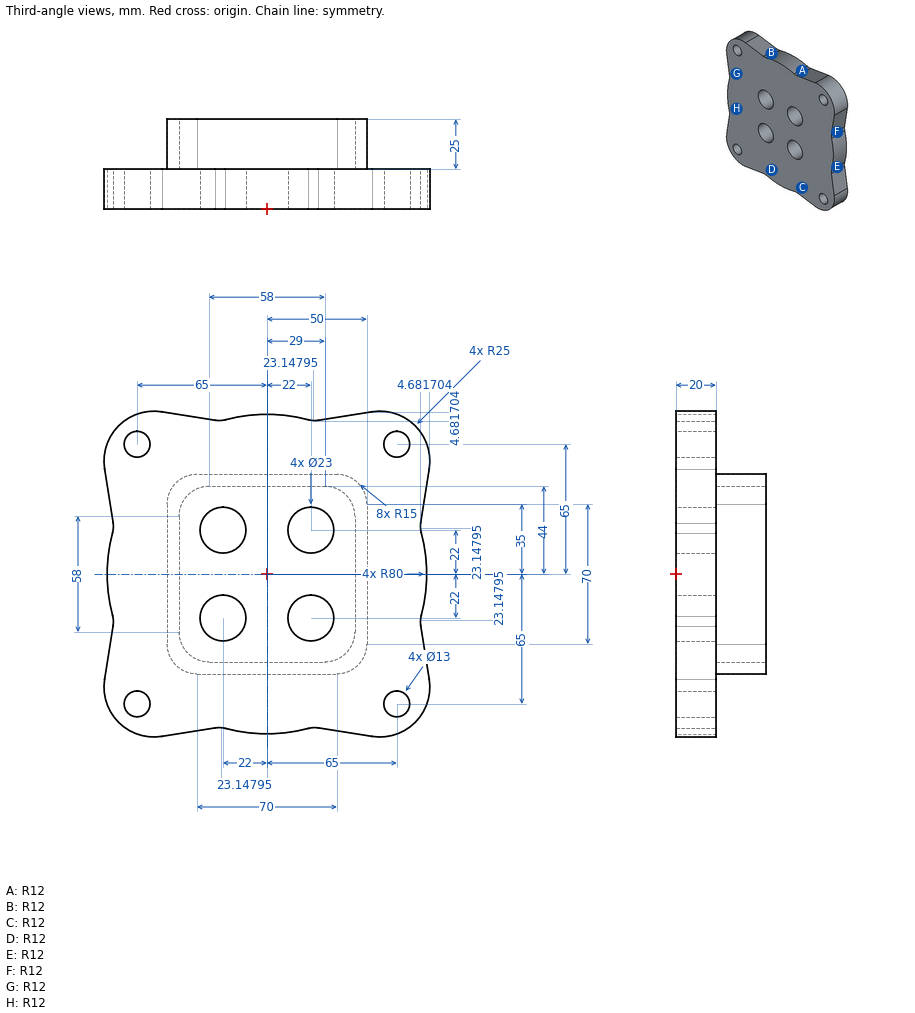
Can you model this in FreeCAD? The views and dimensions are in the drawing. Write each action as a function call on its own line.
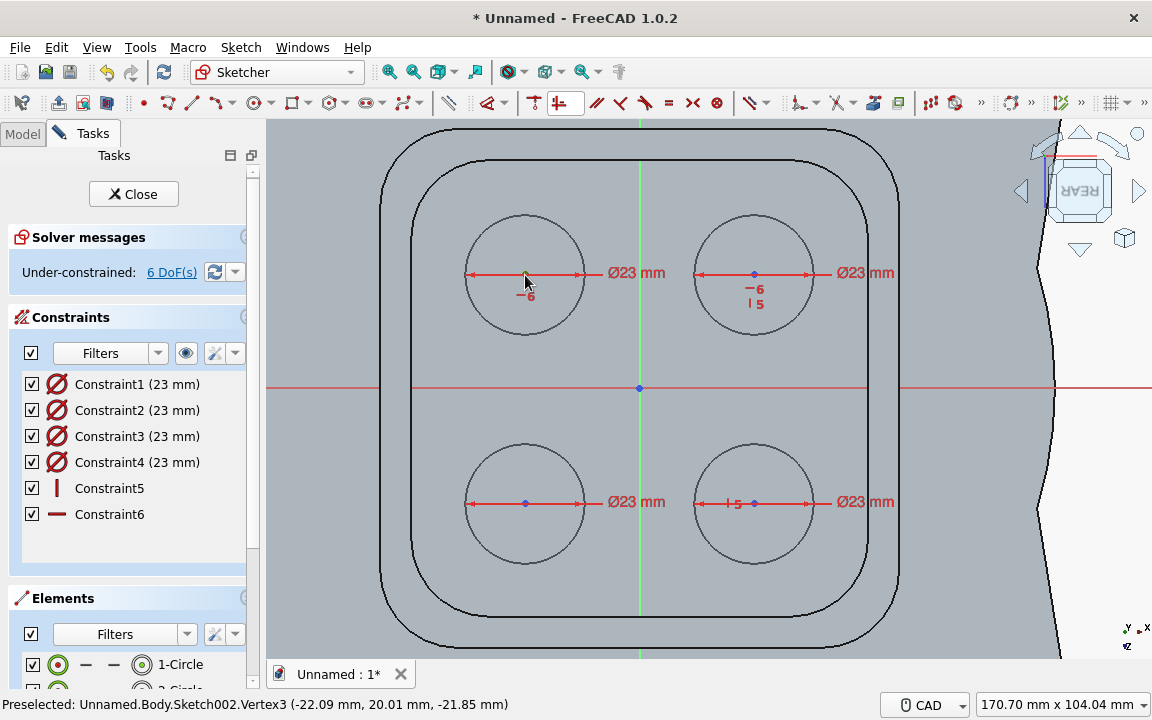
click(525, 504)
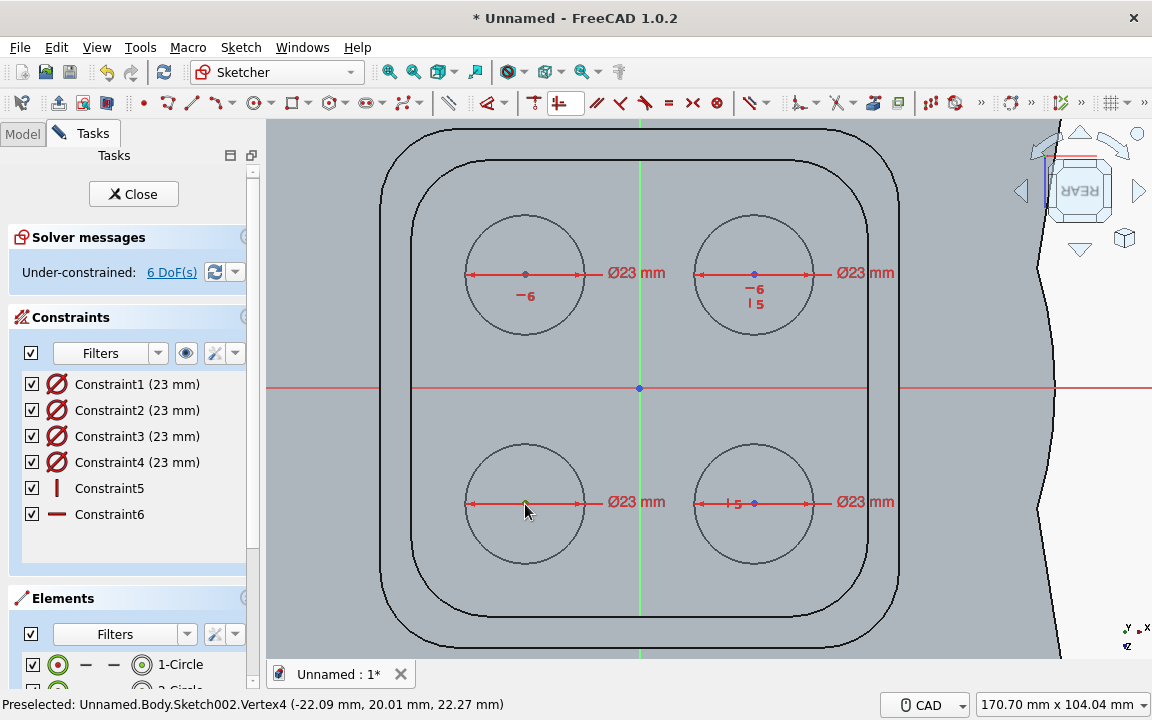
click(578, 104)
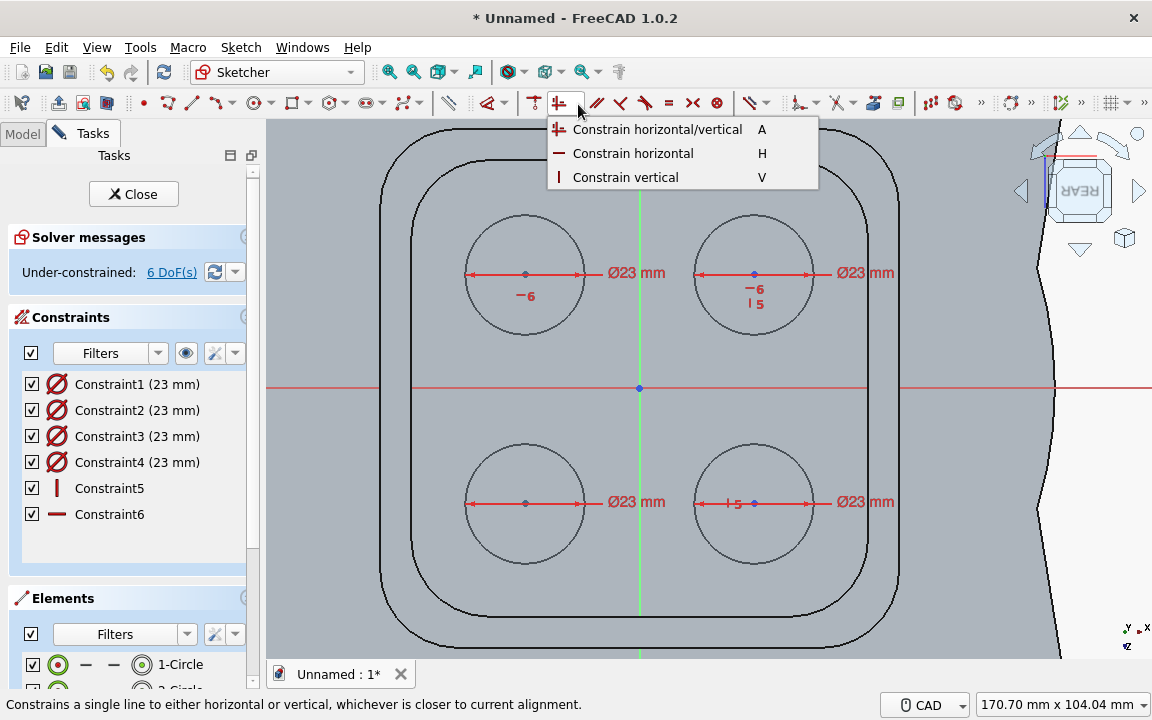
click(683, 177)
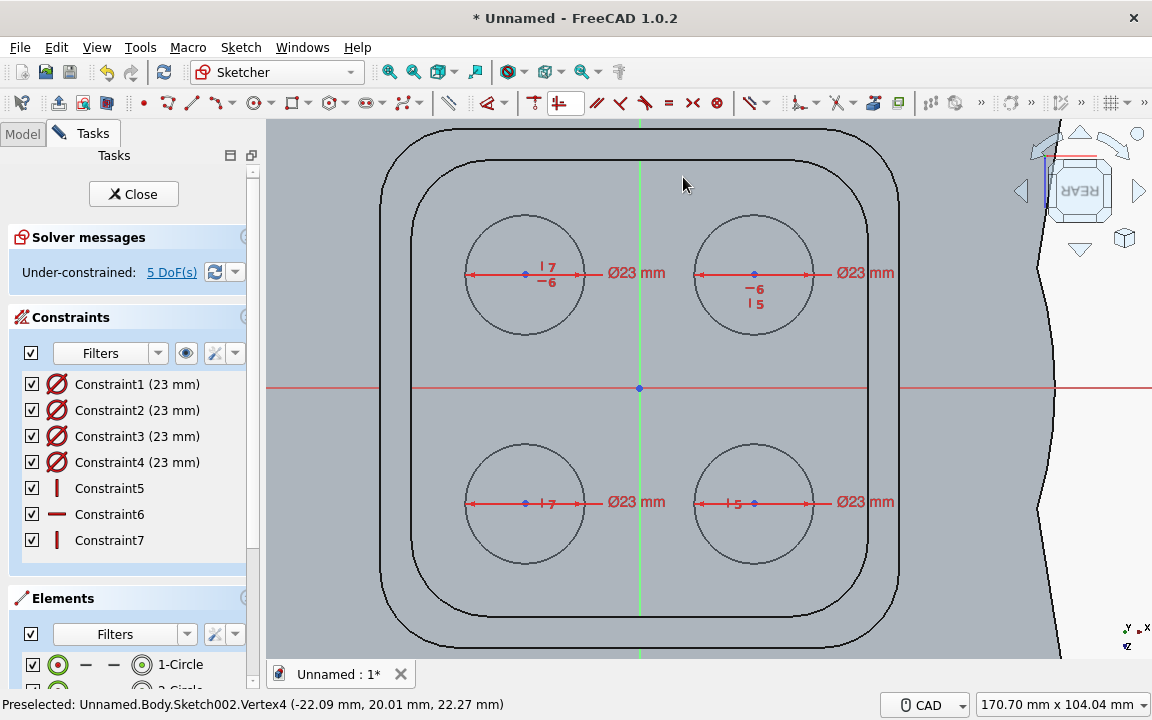
click(754, 504)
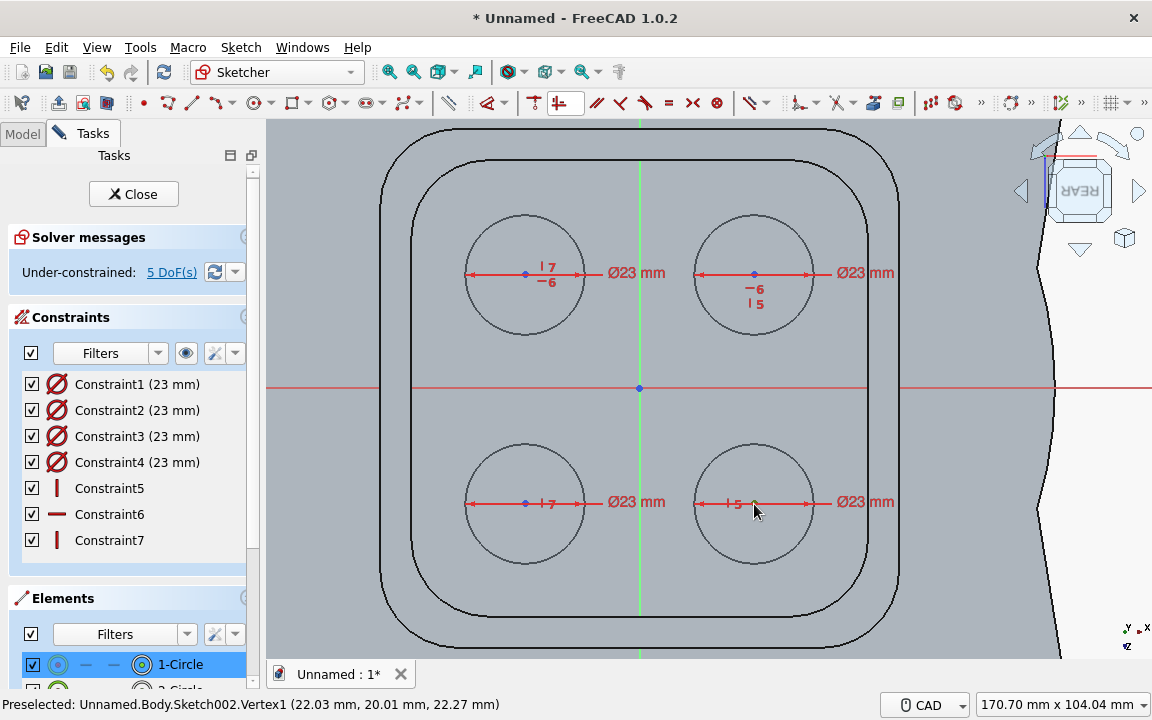
click(525, 504)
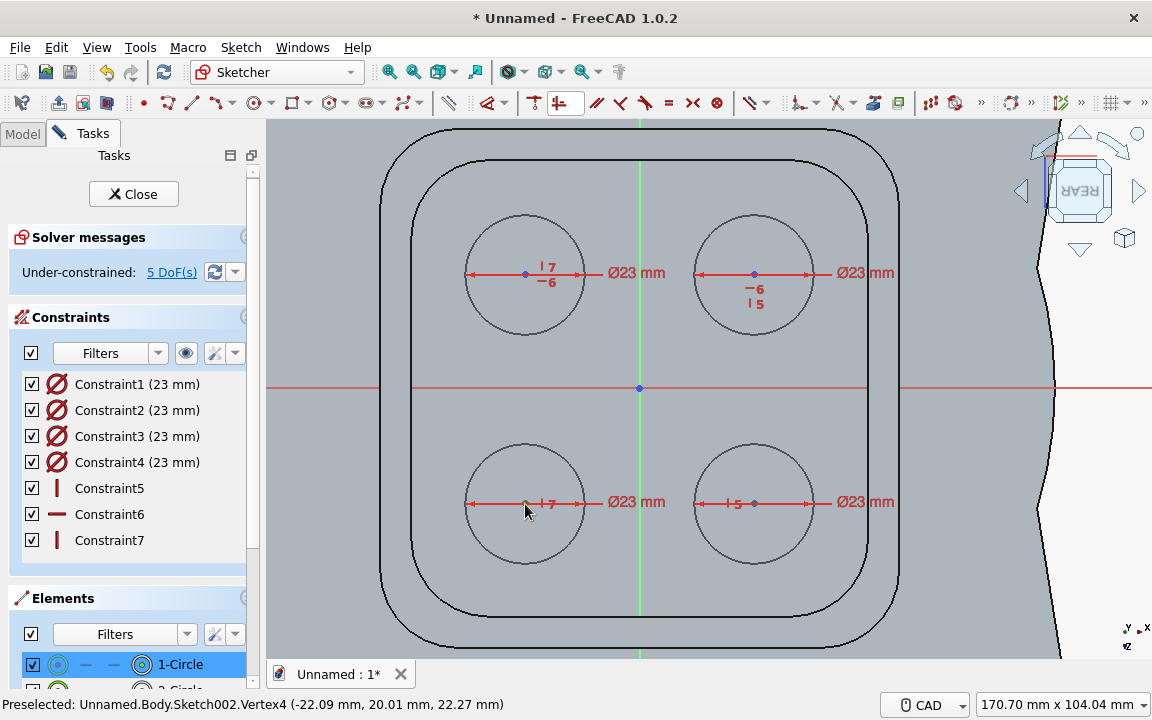
click(578, 104)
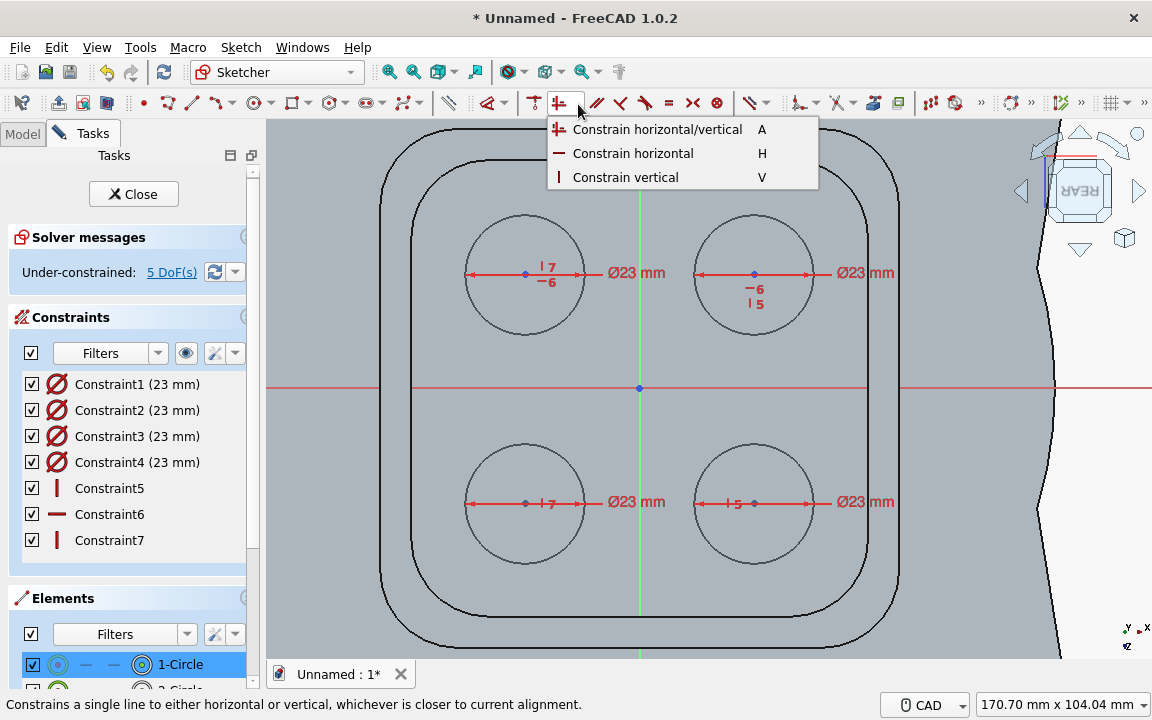
click(683, 153)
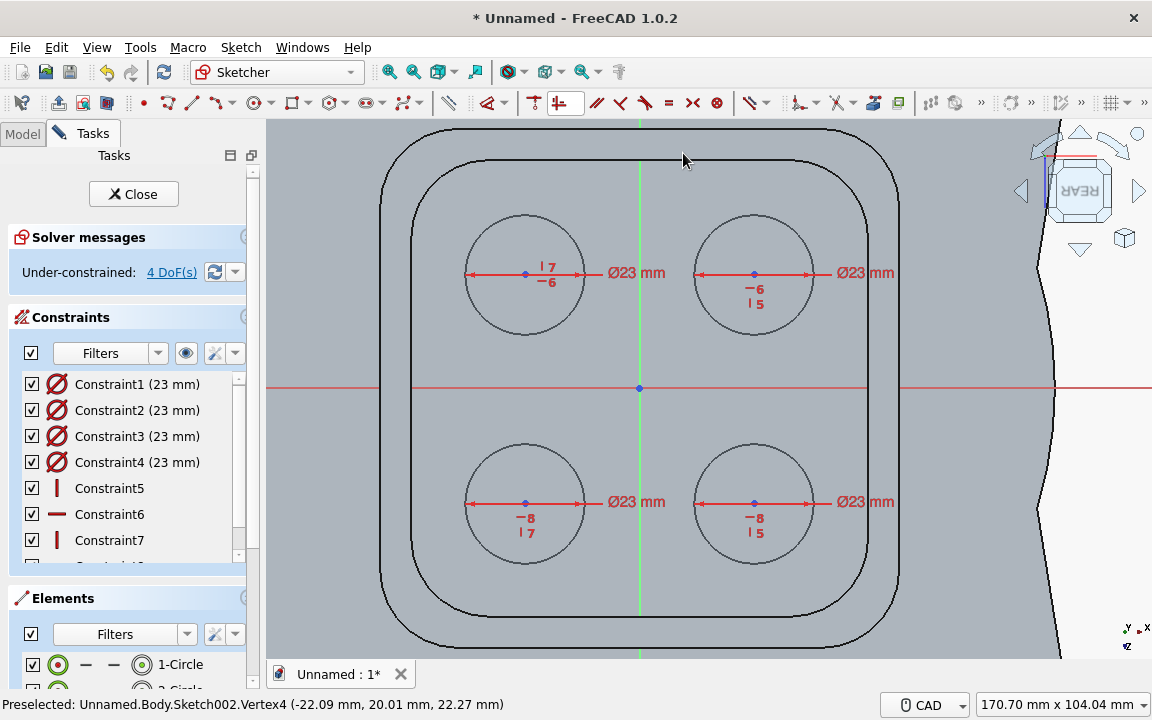
click(488, 104)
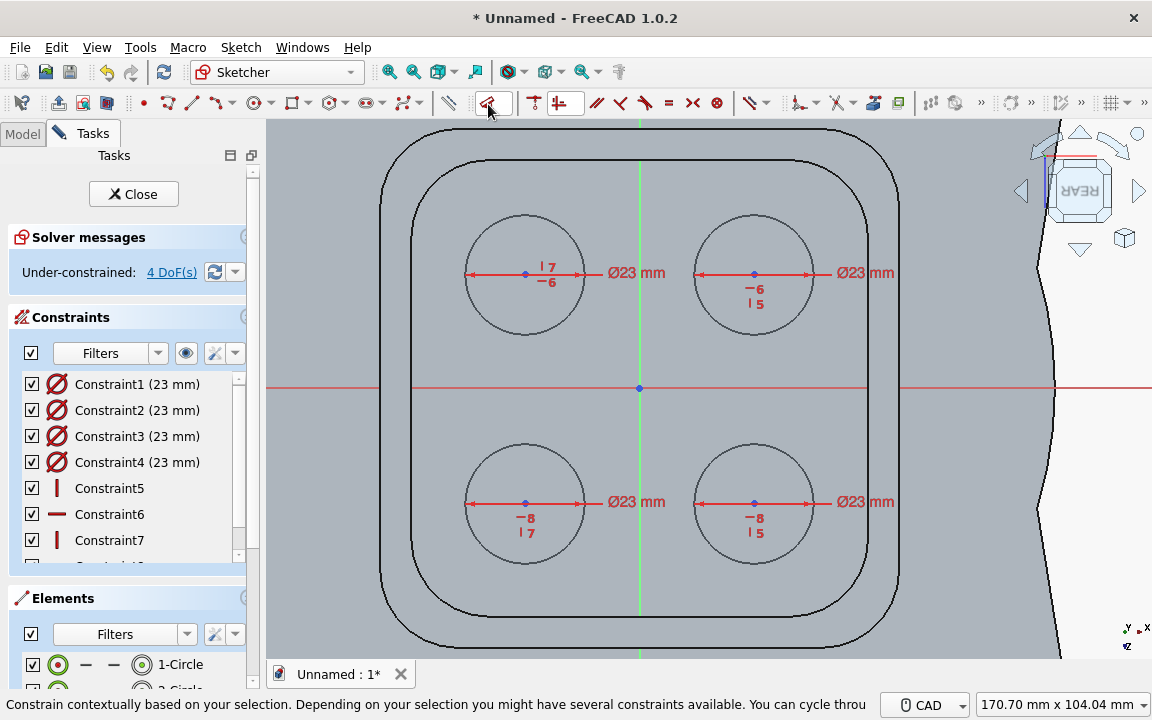
click(754, 504)
click(671, 538)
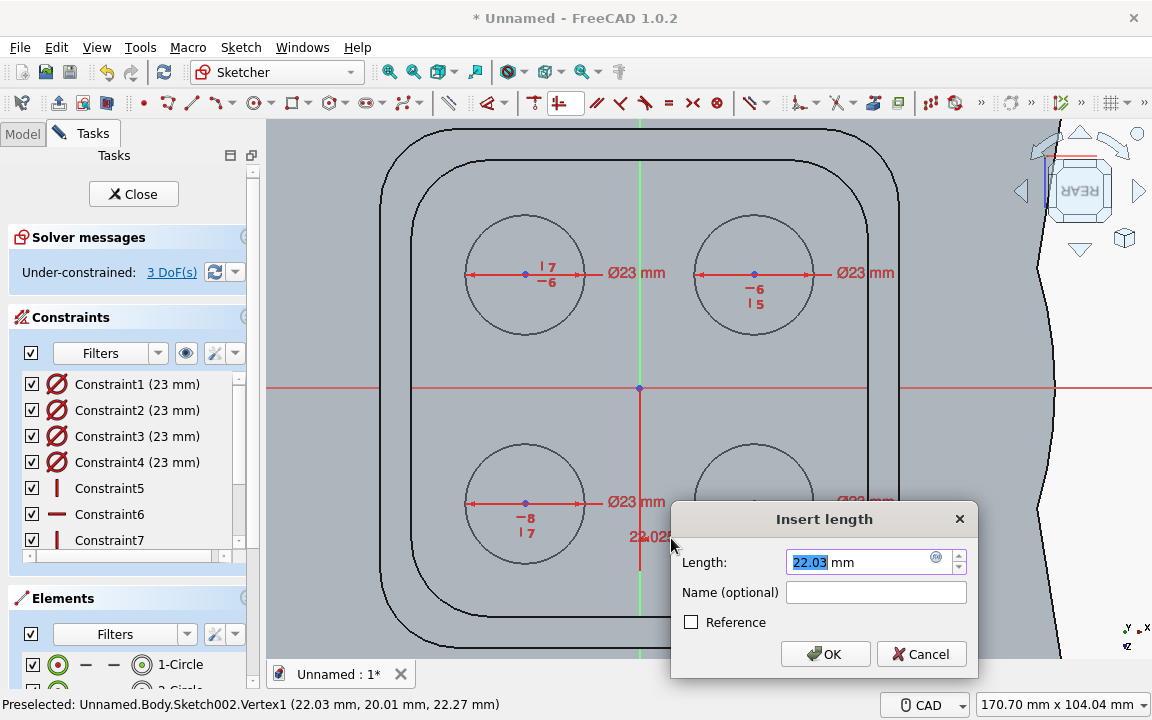
text(22)
key(Return)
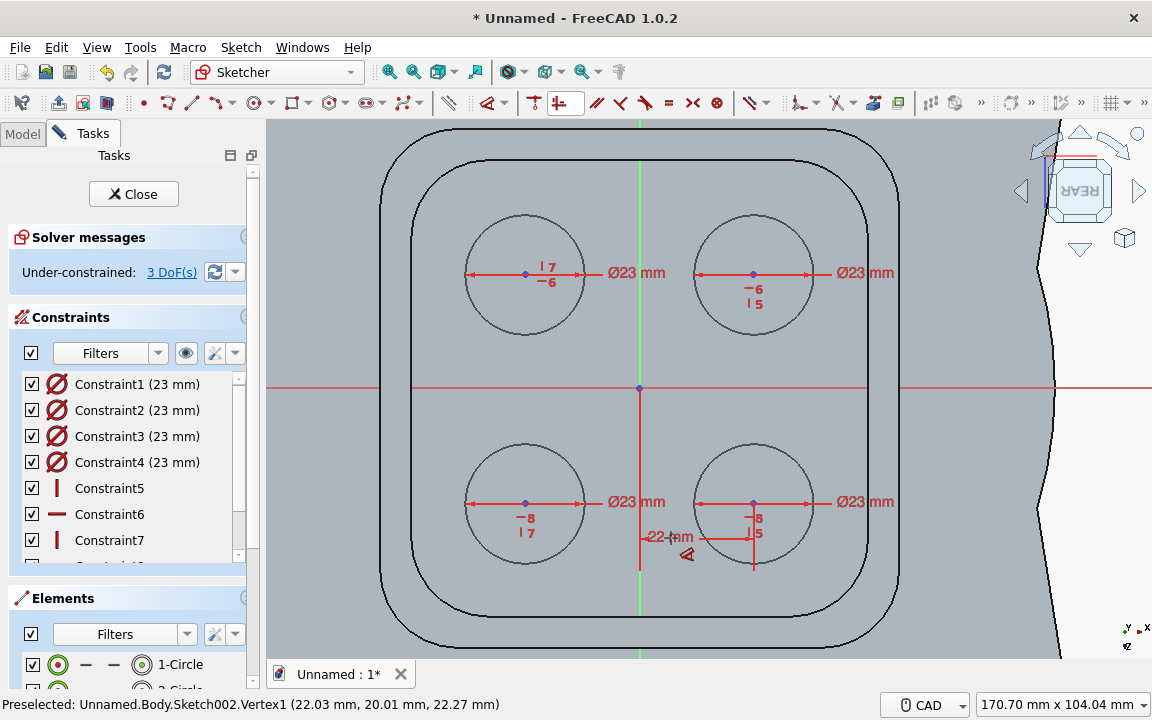
click(754, 504)
click(788, 420)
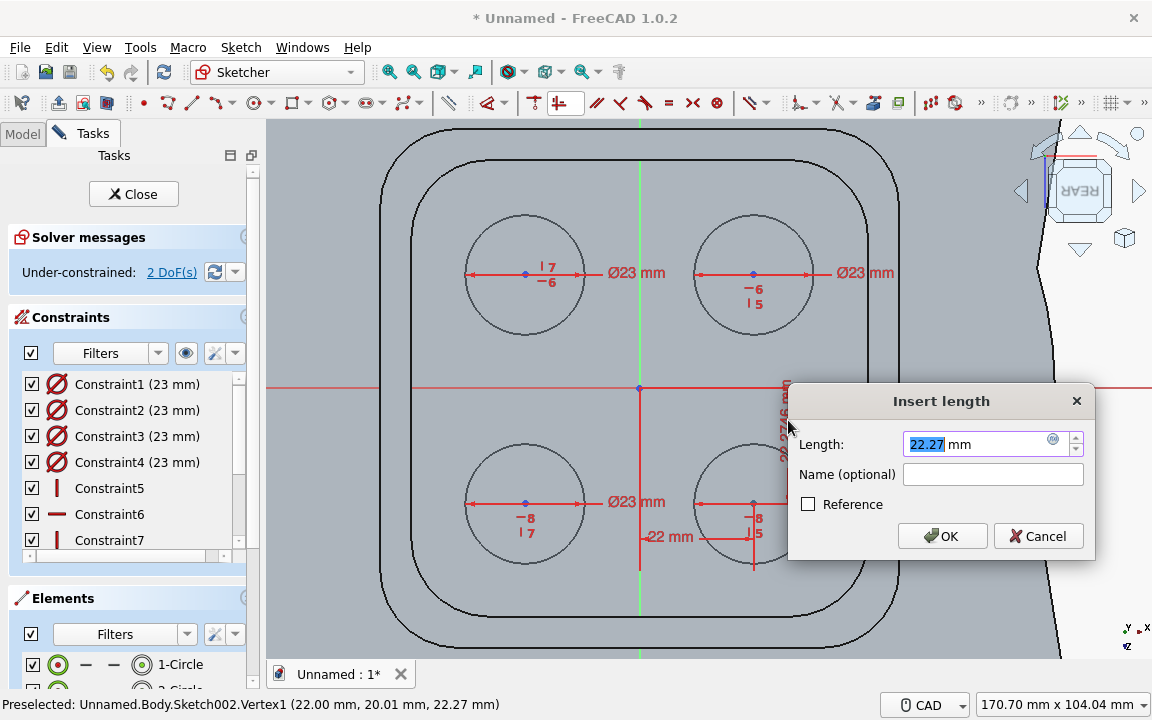
text(22)
key(Return)